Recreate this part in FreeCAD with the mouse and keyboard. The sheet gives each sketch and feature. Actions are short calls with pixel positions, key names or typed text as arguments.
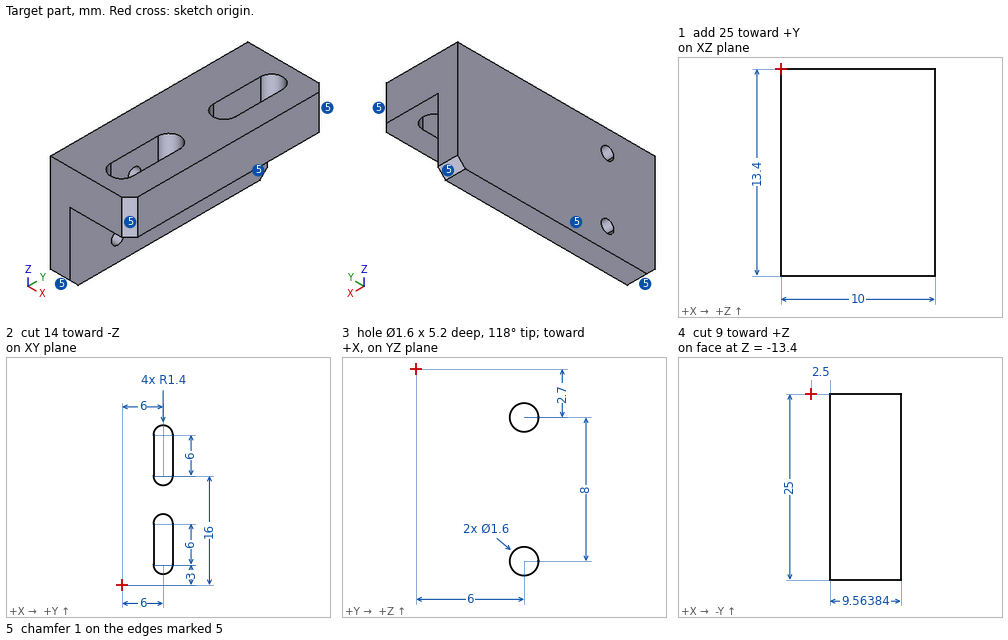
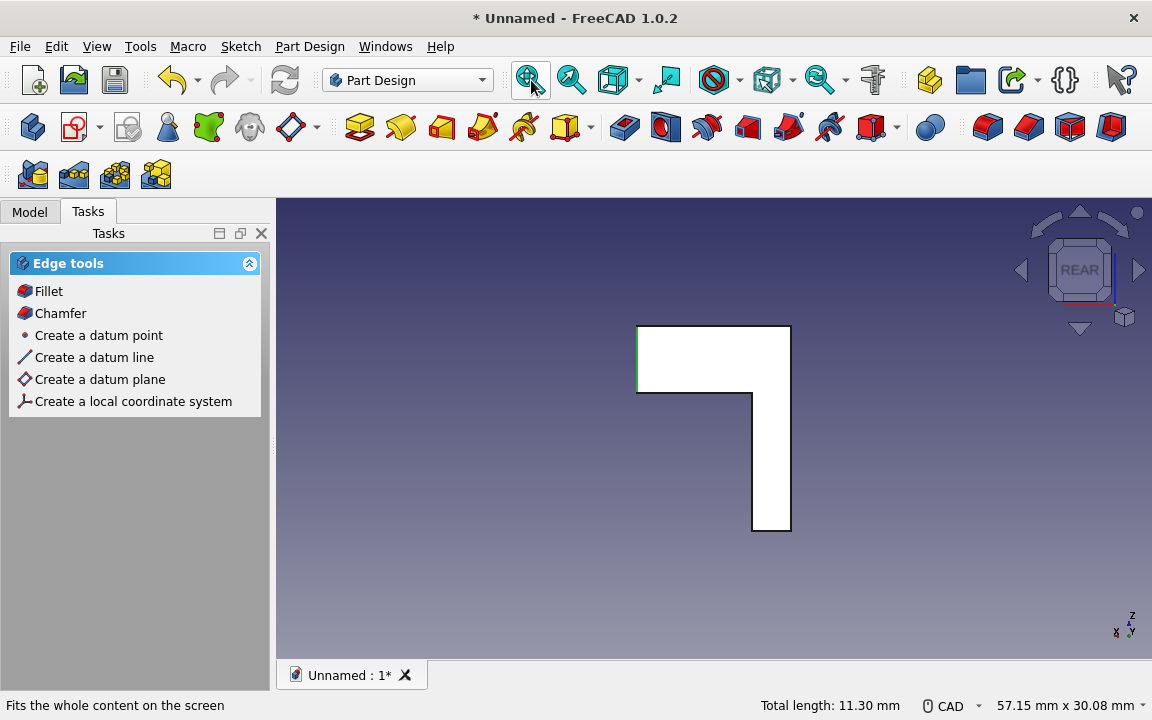
click(771, 530, ctrl)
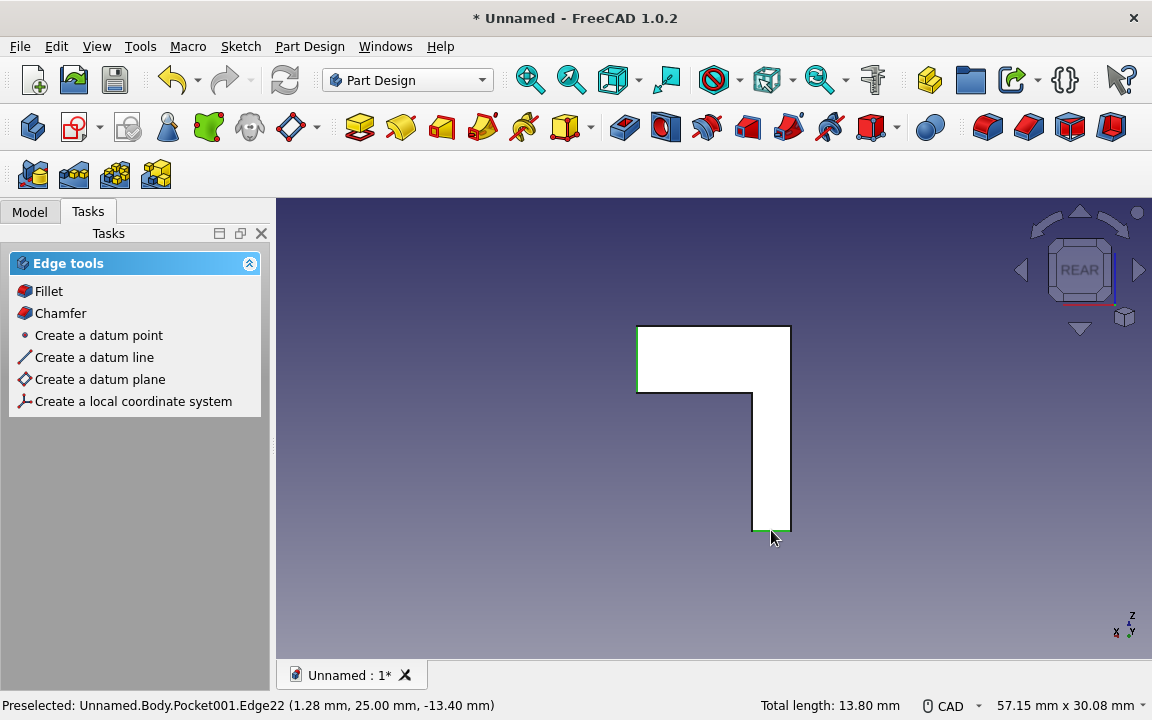
click(1029, 128)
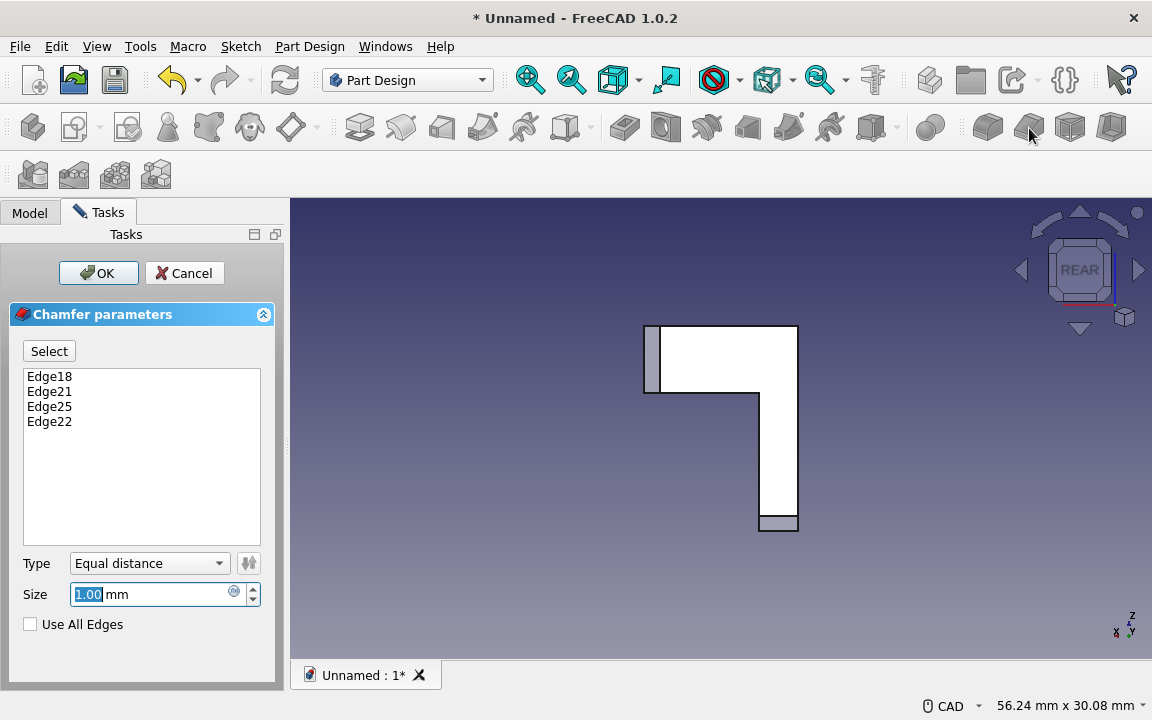
text(1)
key(Tab)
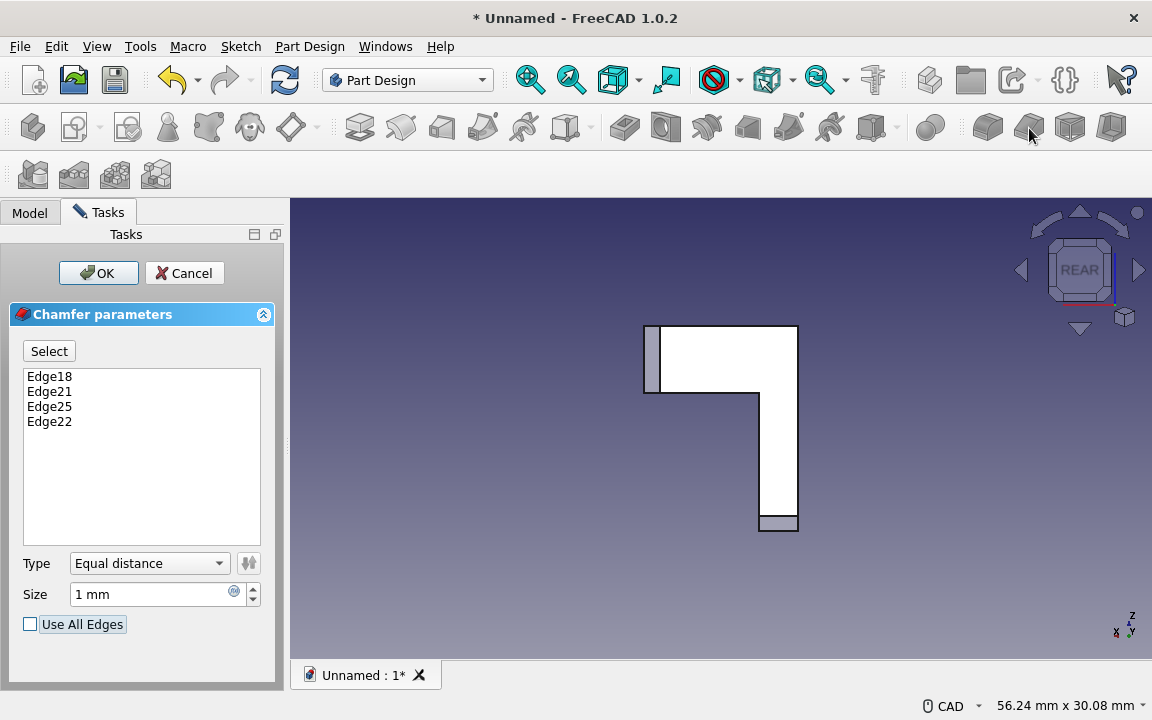
click(99, 273)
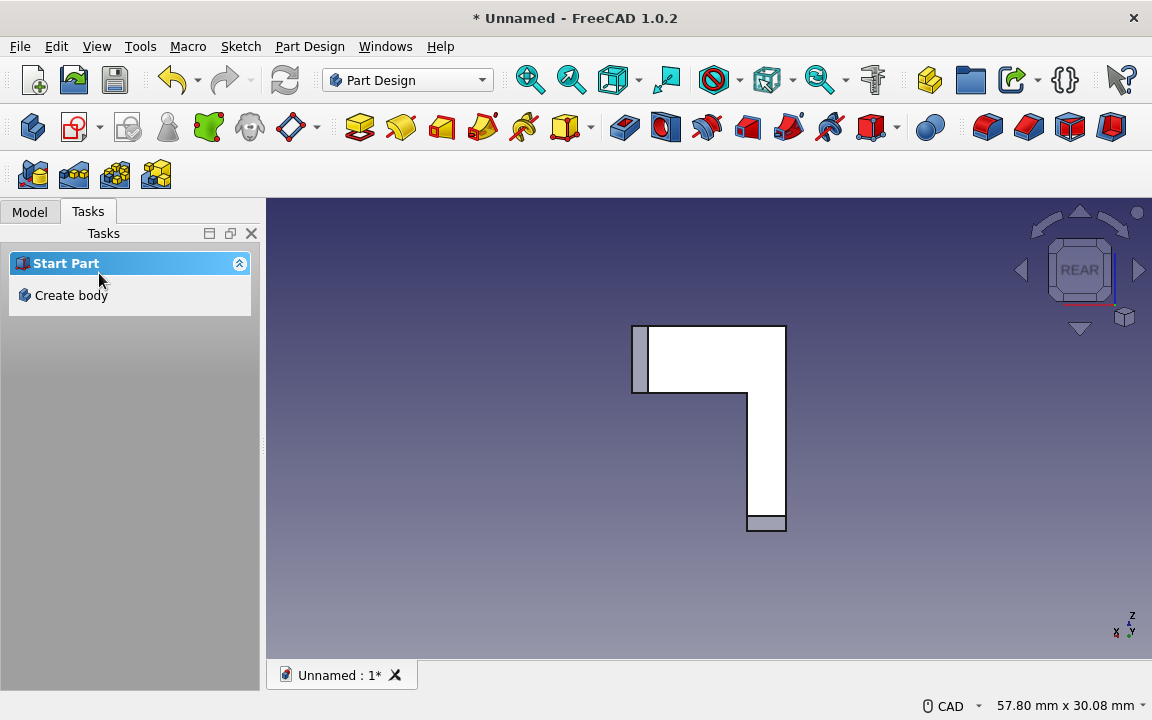
key(0)